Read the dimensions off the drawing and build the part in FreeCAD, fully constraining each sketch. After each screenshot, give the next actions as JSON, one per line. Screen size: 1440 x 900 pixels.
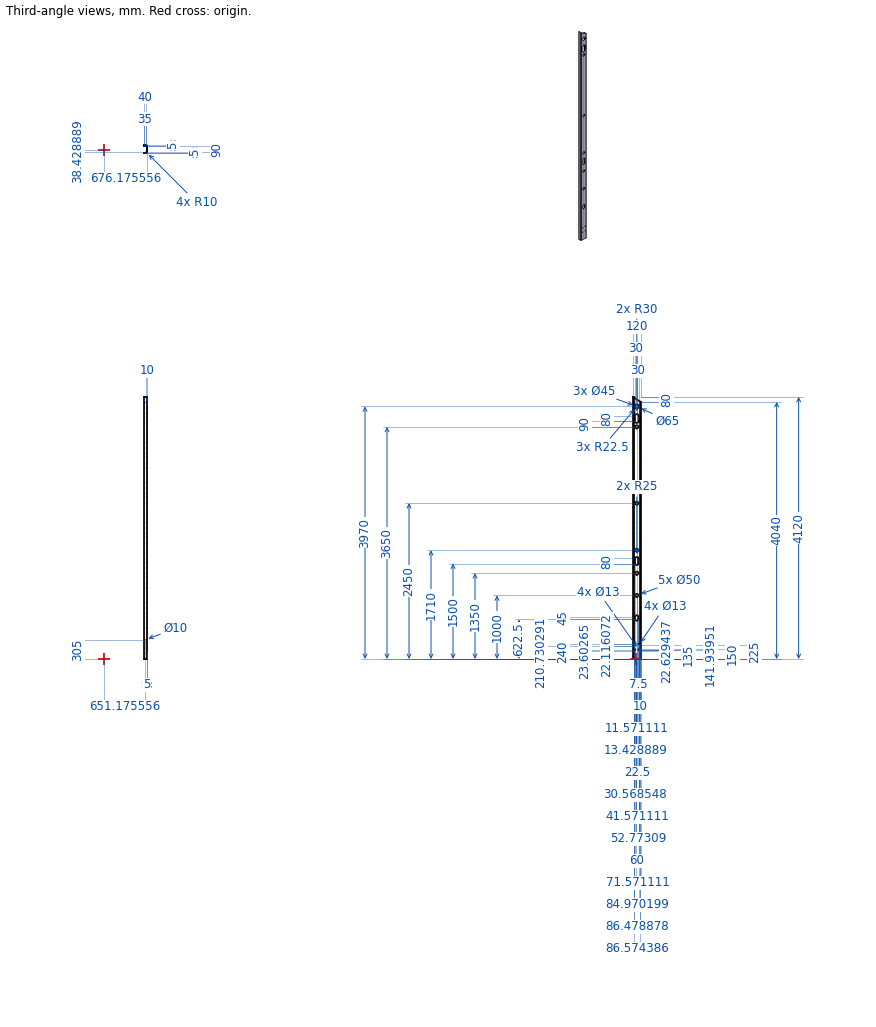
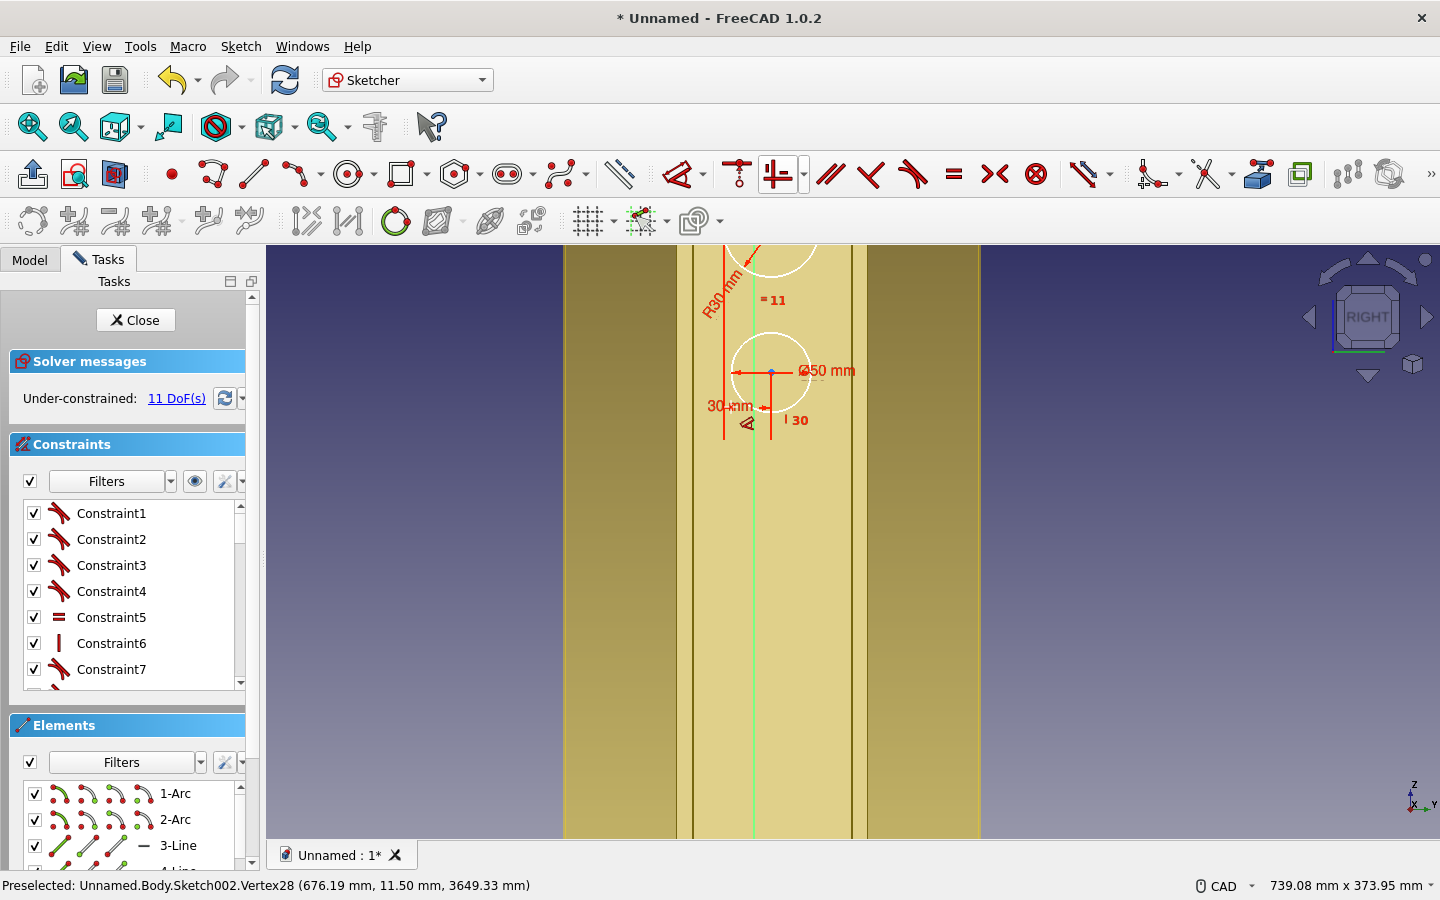
{"action": "scroll", "coordinate": [785, 383], "scroll_direction": "down", "scroll_amount": 14}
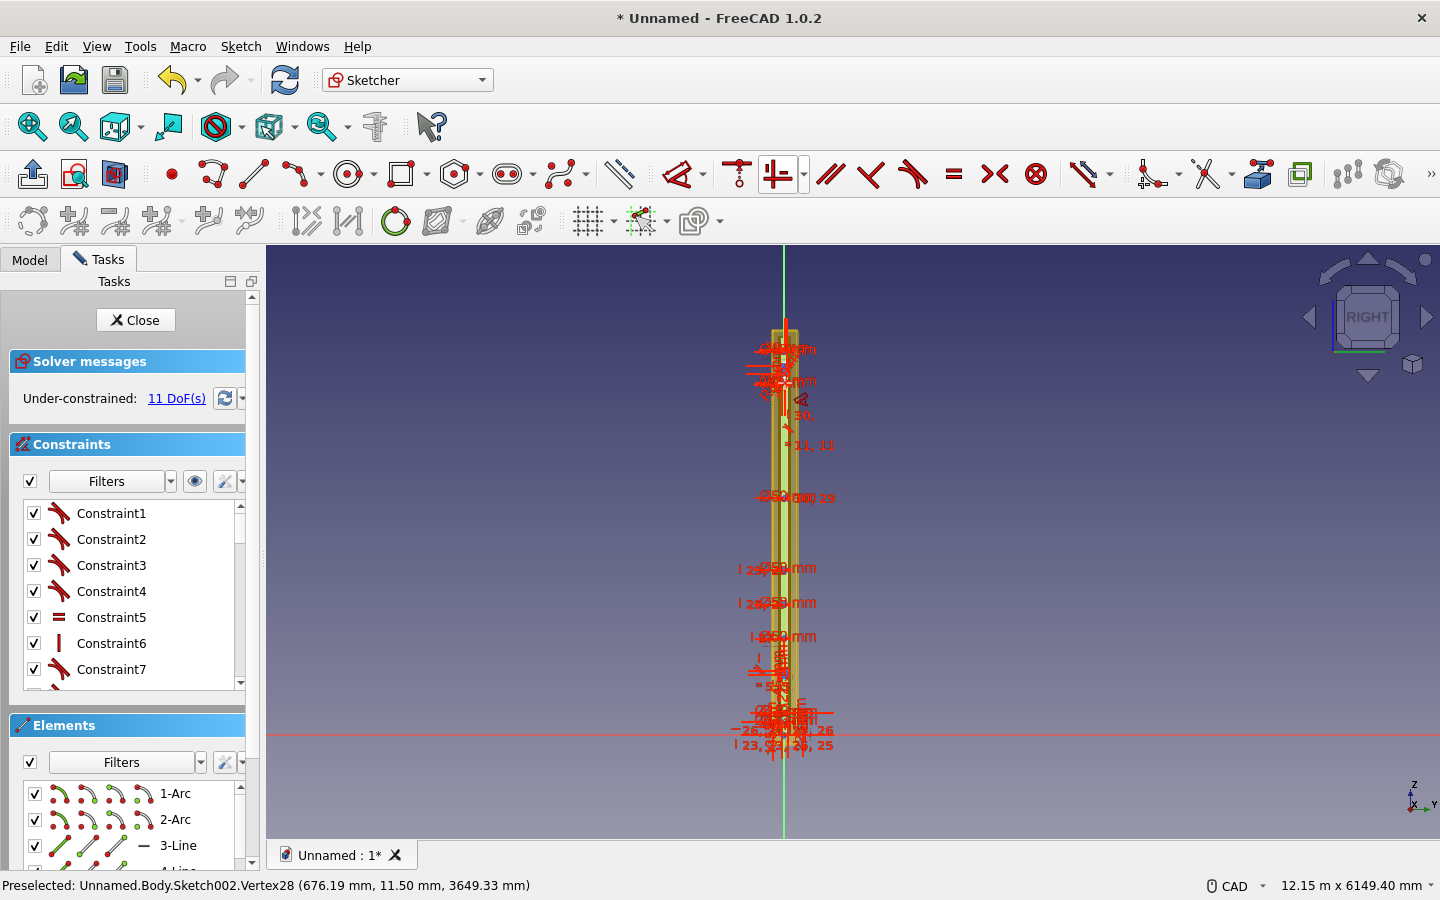
{"action": "scroll", "coordinate": [782, 374], "scroll_direction": "up", "scroll_amount": 8}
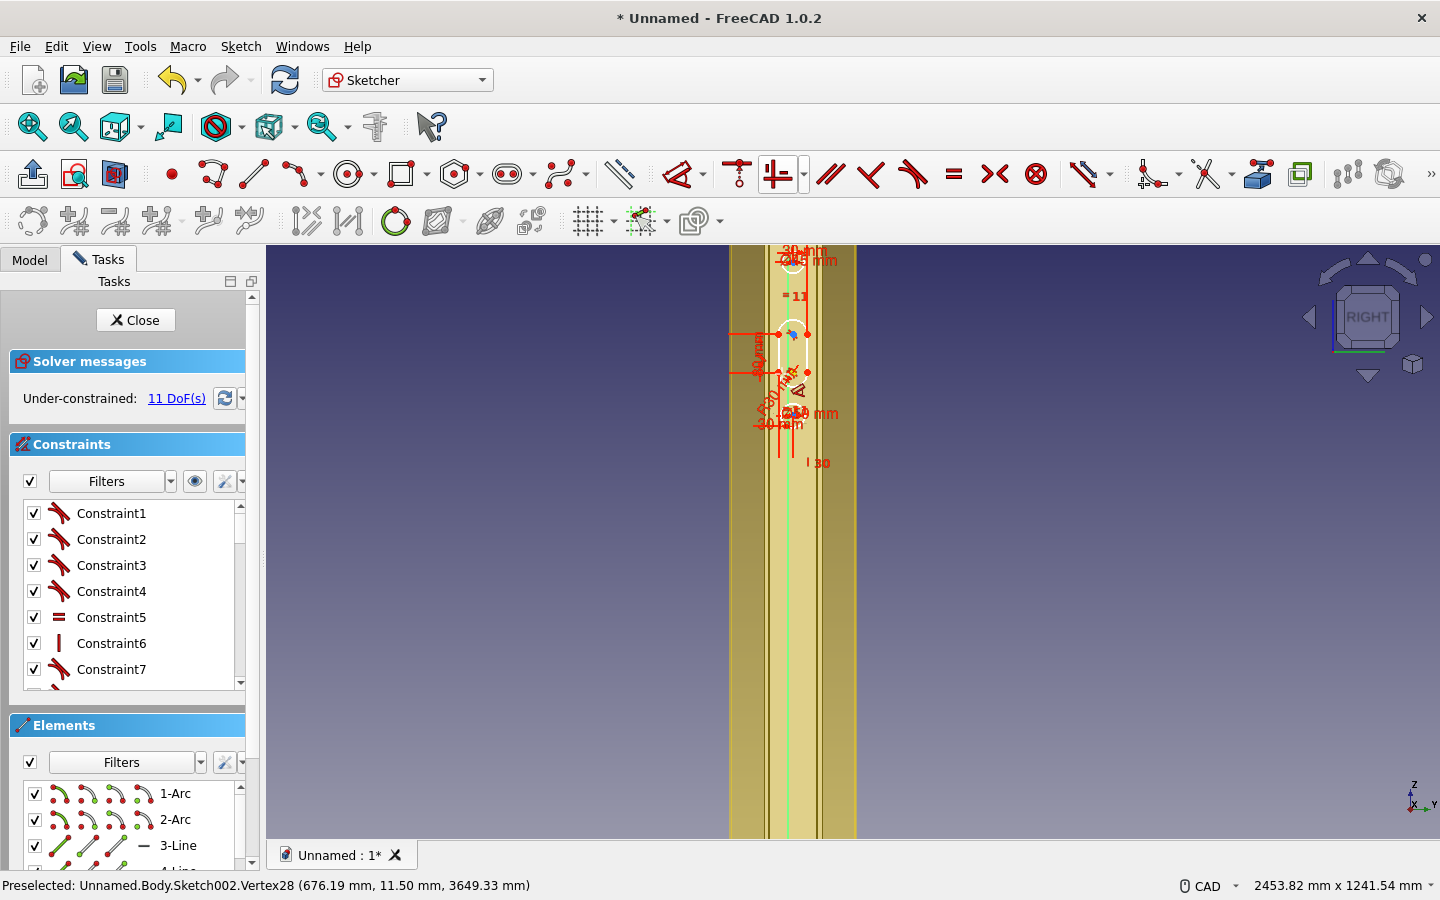
{"action": "left_click", "coordinate": [779, 373]}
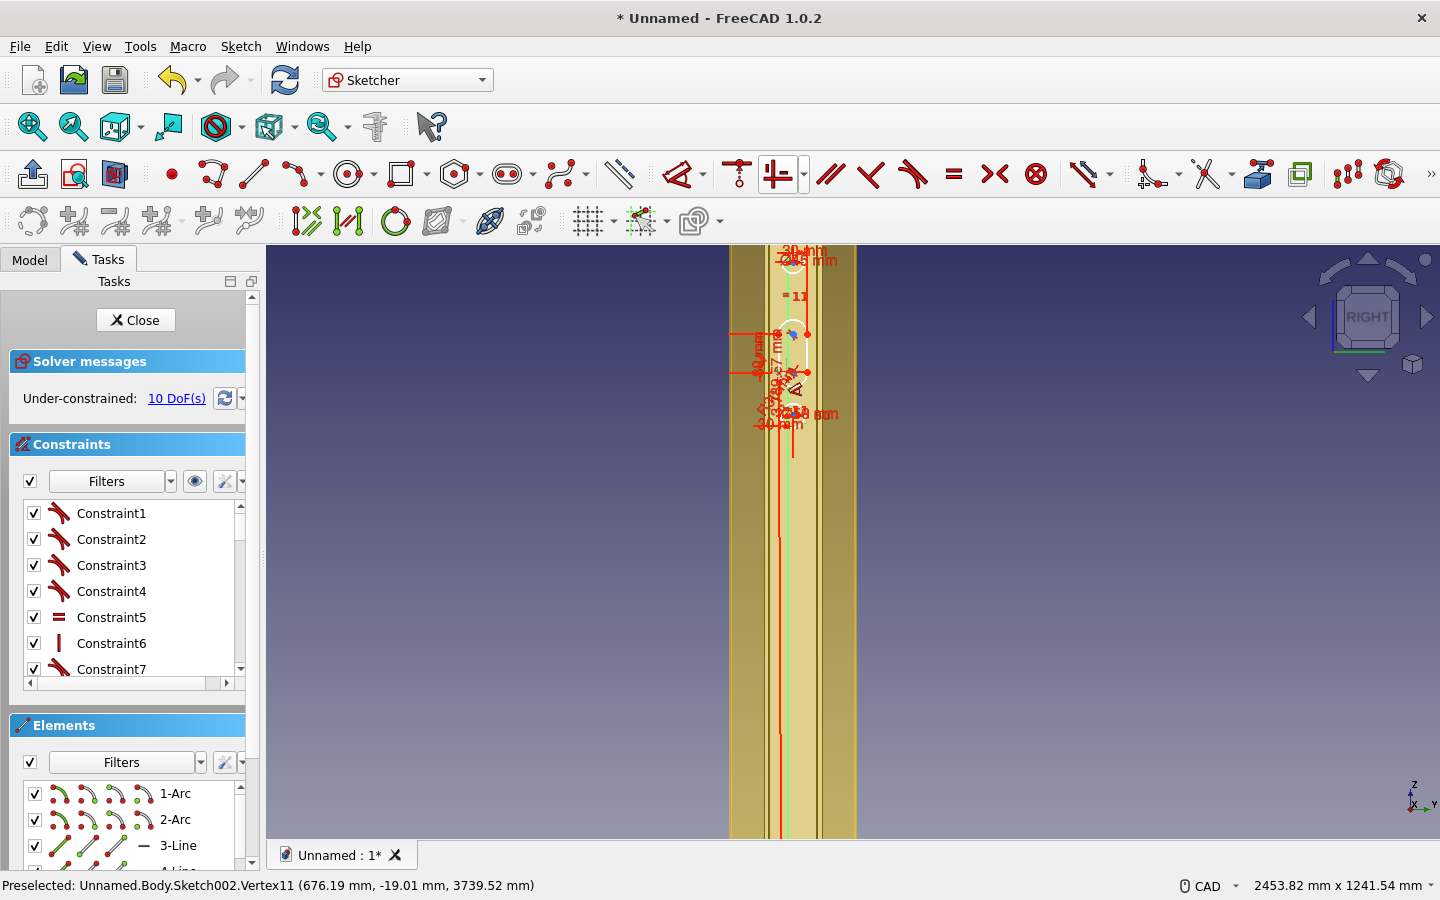
{"action": "left_click", "coordinate": [793, 416]}
{"action": "left_click", "coordinate": [851, 394]}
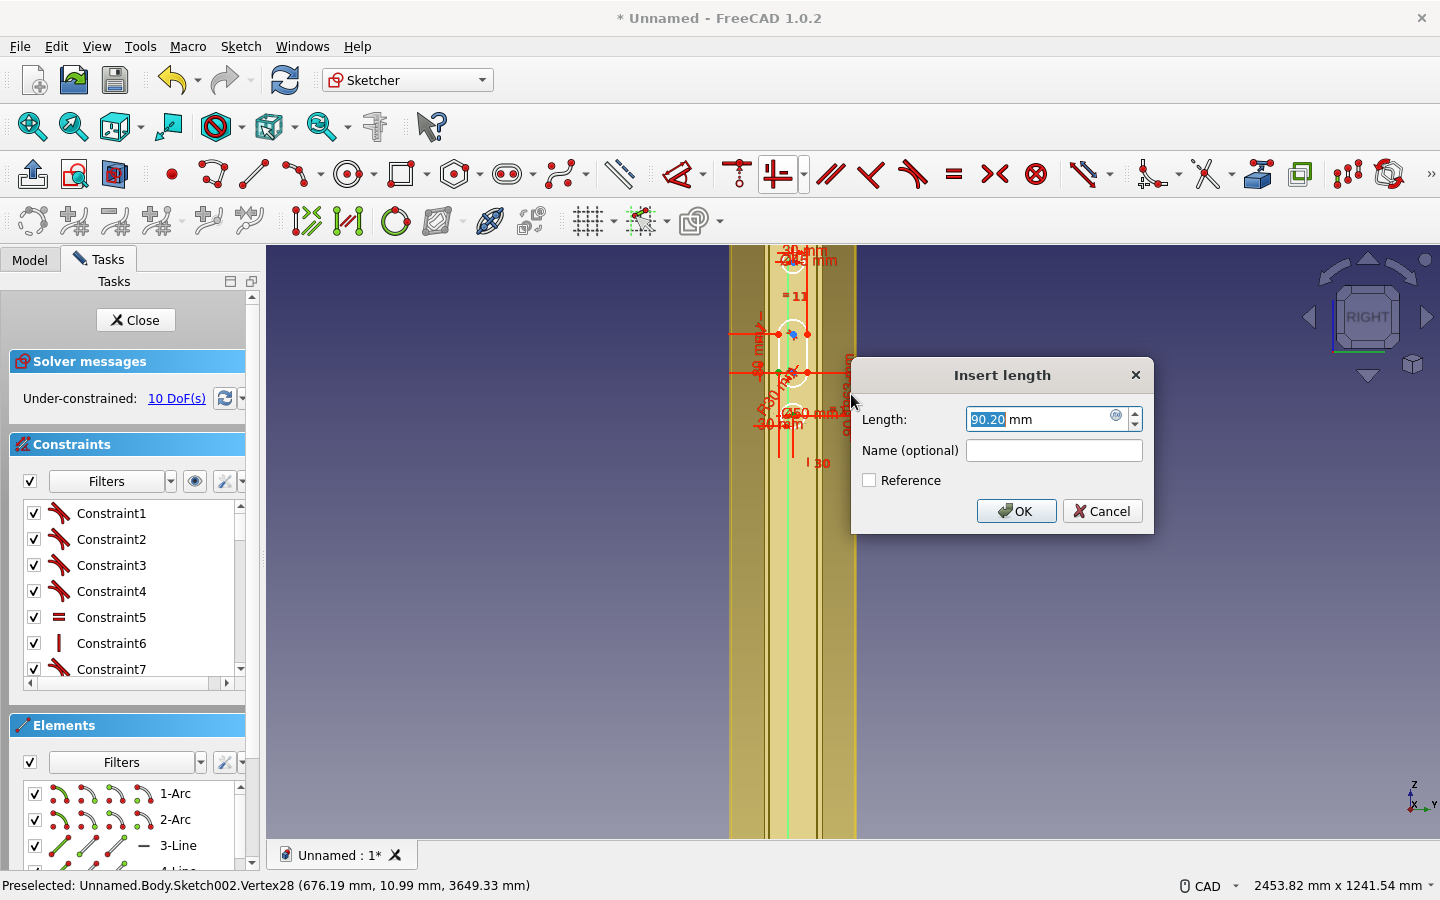
{"action": "type", "text": "90"}
{"action": "key", "text": "Return"}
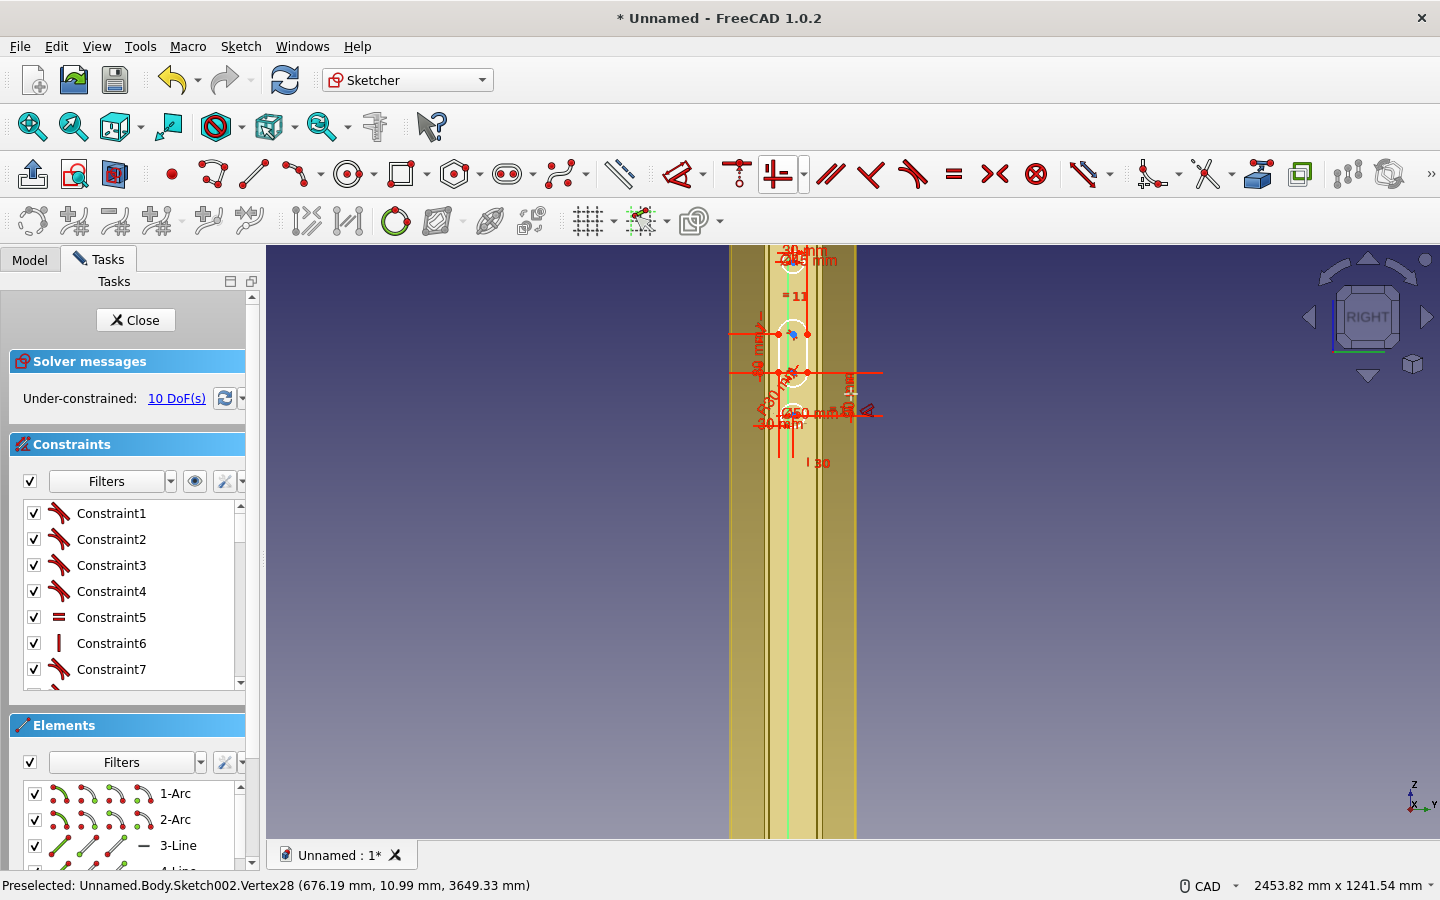
{"action": "scroll", "coordinate": [782, 374], "scroll_direction": "down", "scroll_amount": 8}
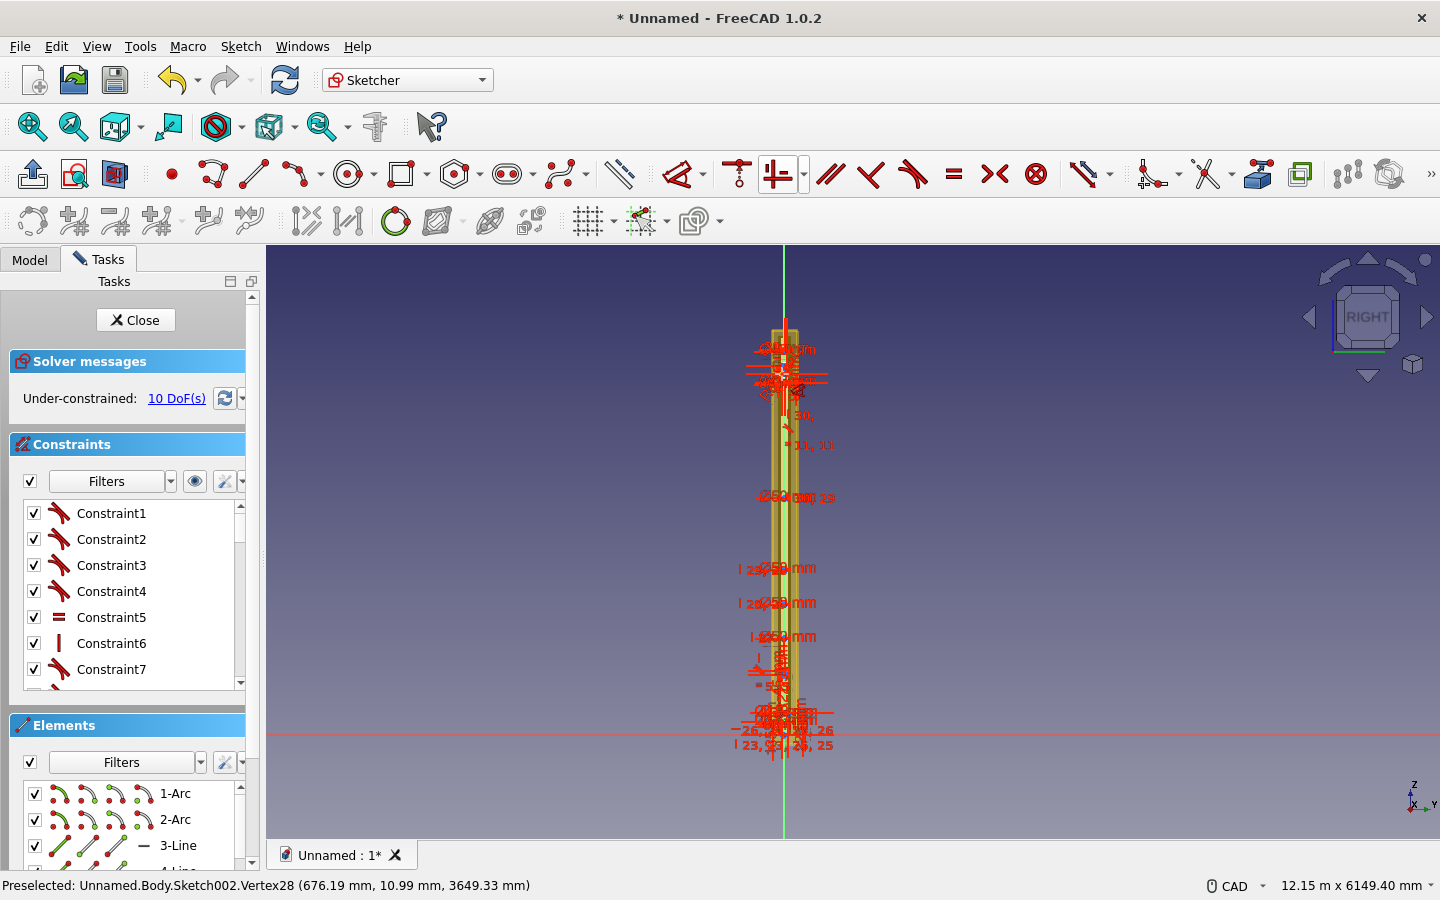
{"action": "left_click", "coordinate": [785, 639]}
{"action": "left_click", "coordinate": [702, 687]}